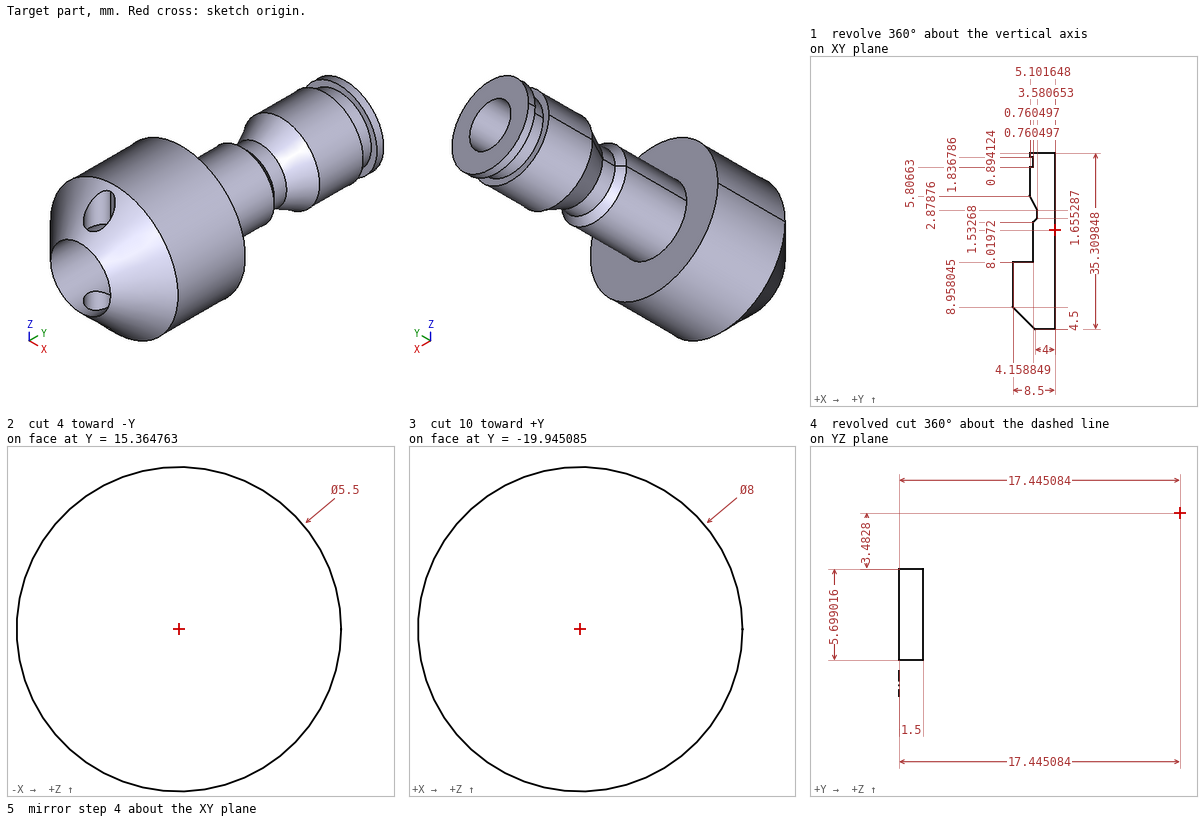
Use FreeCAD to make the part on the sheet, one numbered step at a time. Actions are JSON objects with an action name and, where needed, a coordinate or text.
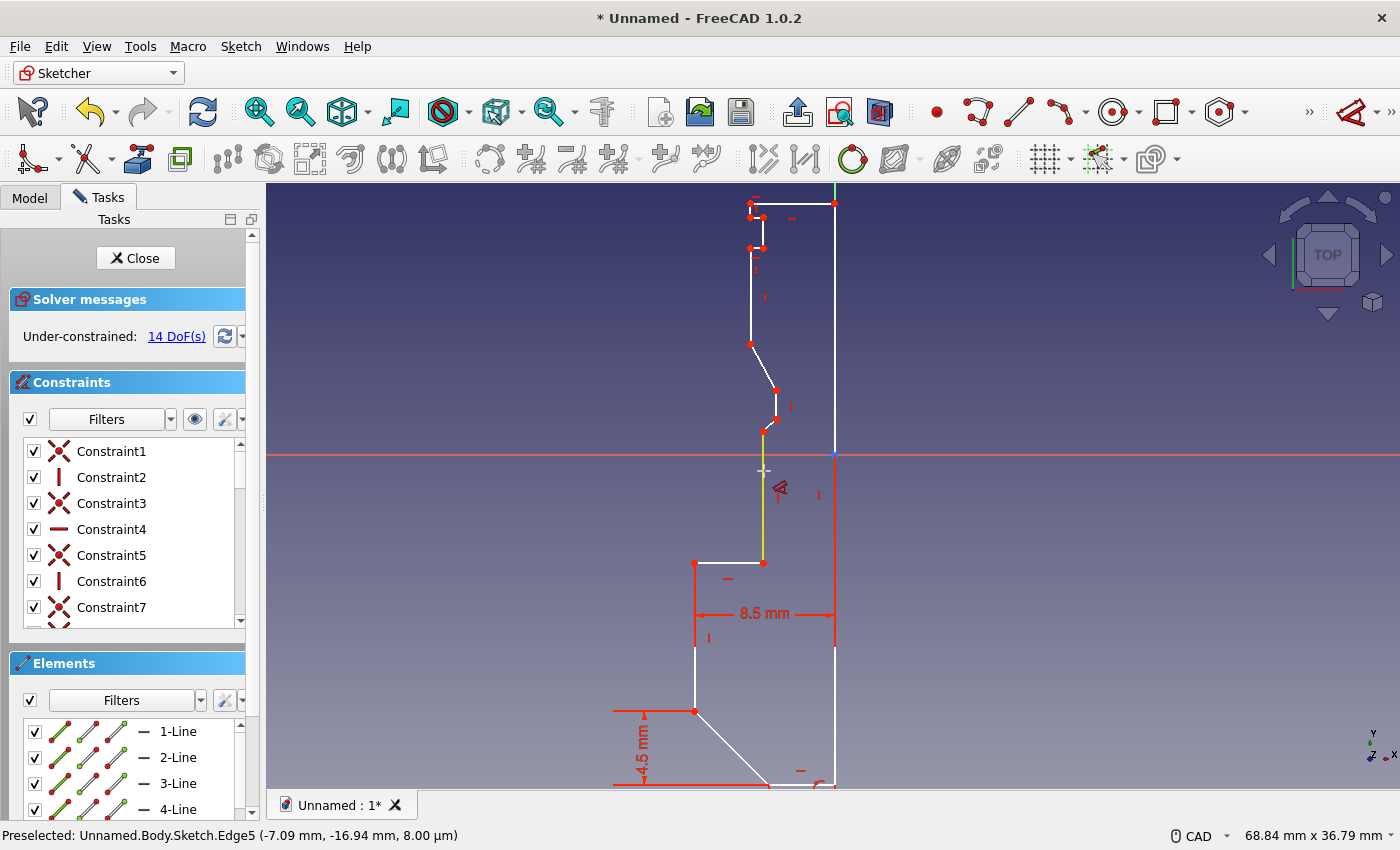
{"action": "left_click", "coordinate": [763, 471]}
{"action": "left_click", "coordinate": [729, 497]}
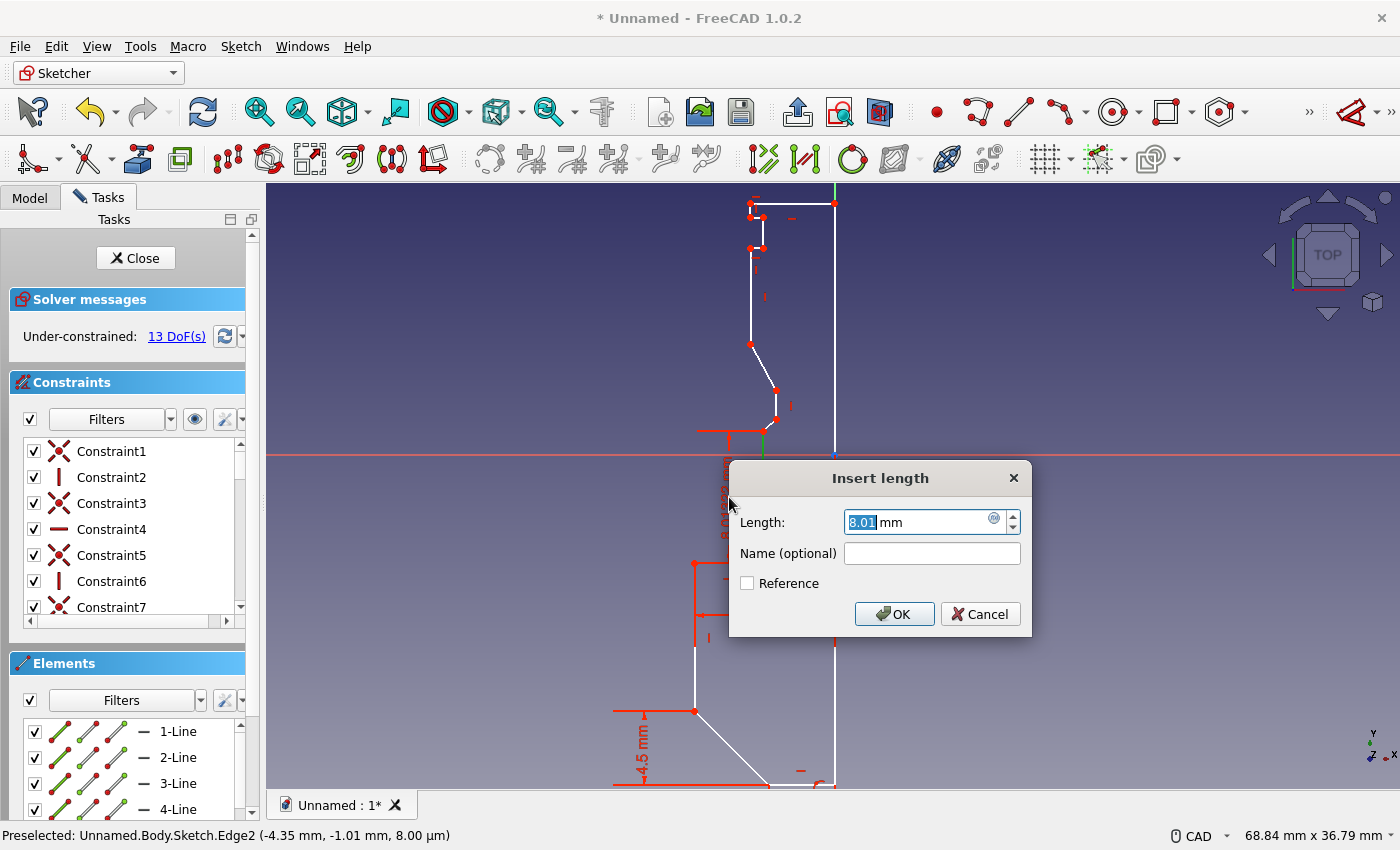
{"action": "type", "text": "8.01972"}
{"action": "key", "text": "Return"}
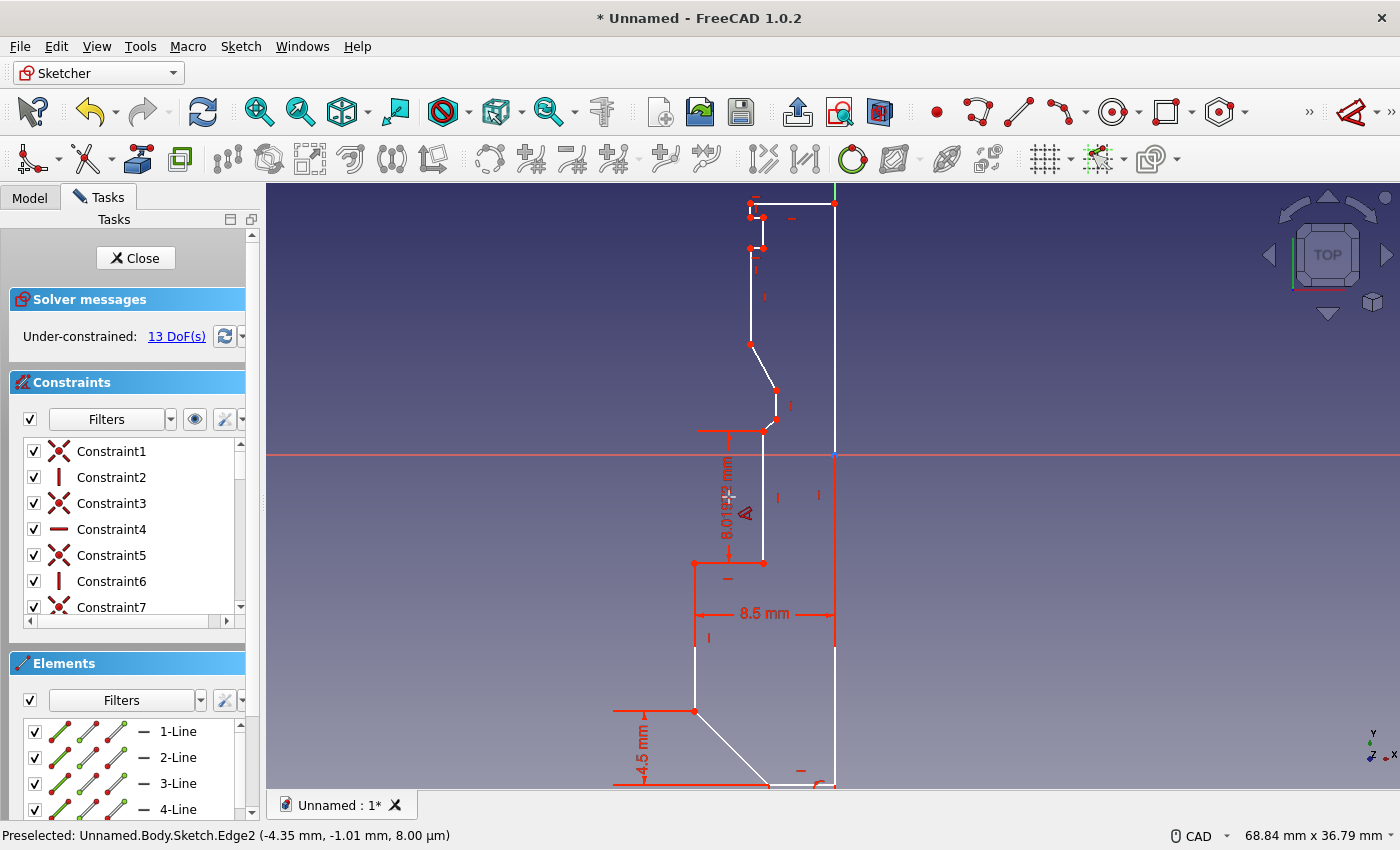
{"action": "left_click", "coordinate": [751, 277]}
{"action": "left_click", "coordinate": [717, 296]}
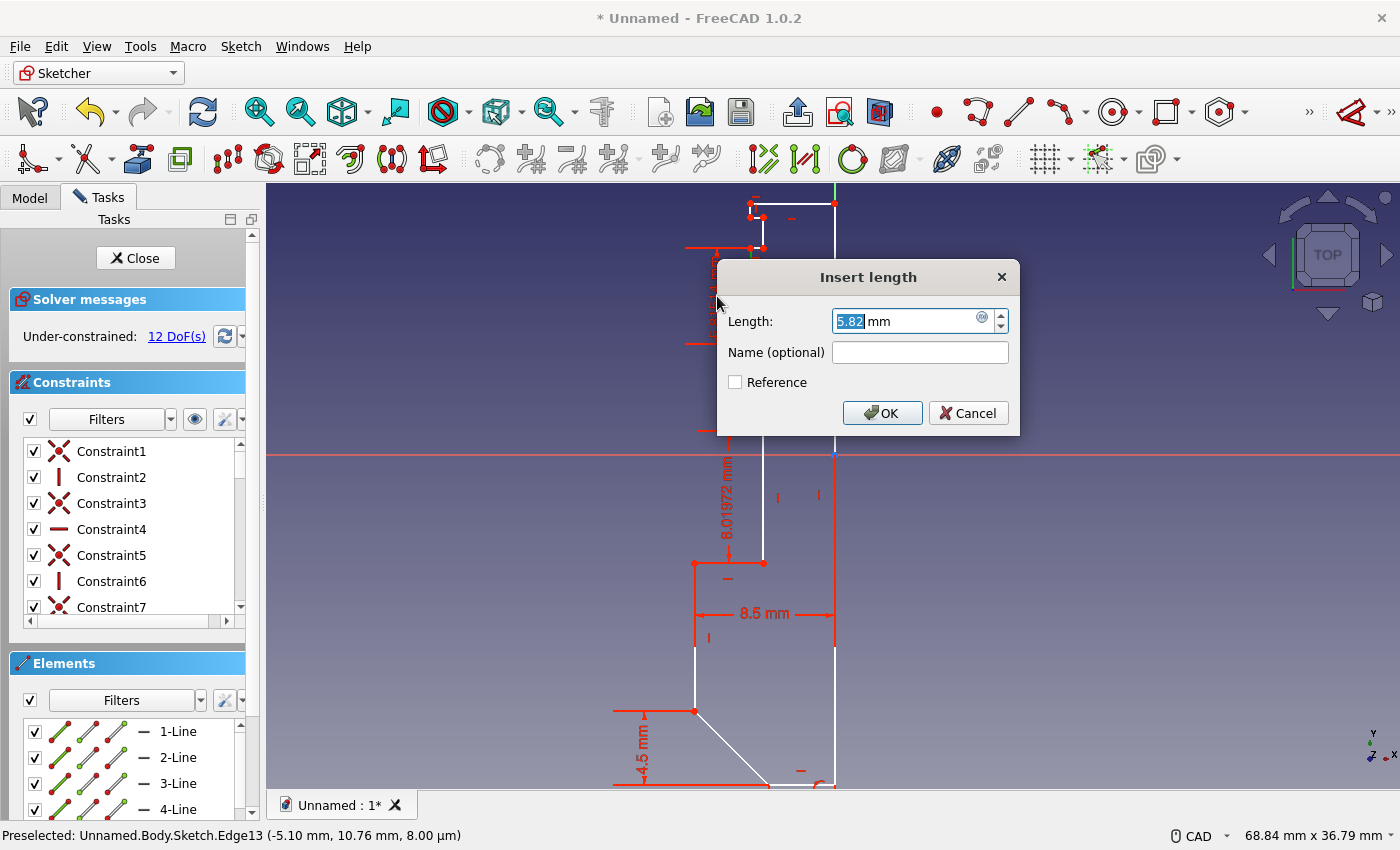
{"action": "type", "text": "5.80663"}
{"action": "key", "text": "Return"}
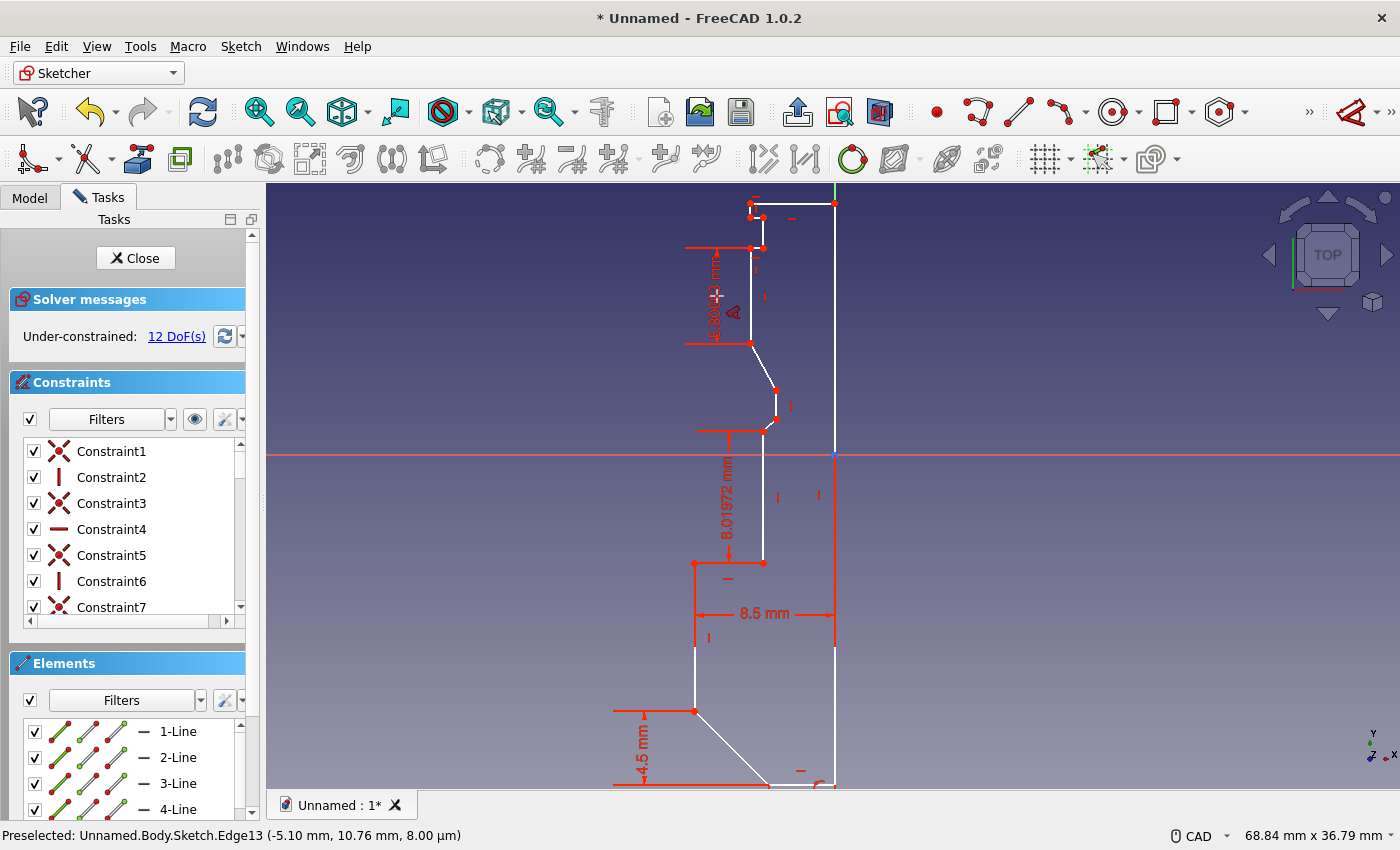
{"action": "left_click", "coordinate": [743, 563]}
{"action": "left_click", "coordinate": [729, 529]}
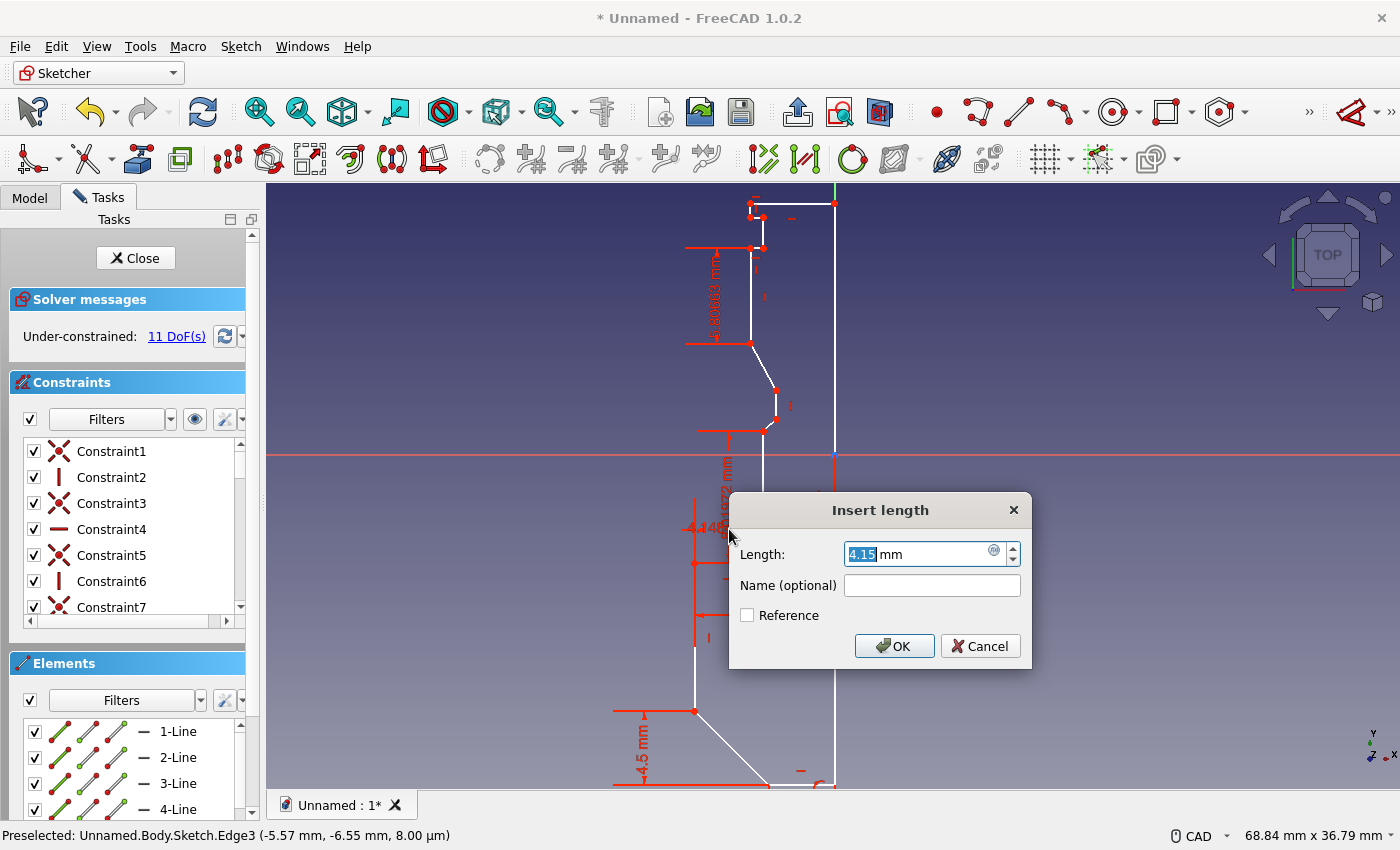
{"action": "type", "text": "4.158849"}
{"action": "key", "text": "Return"}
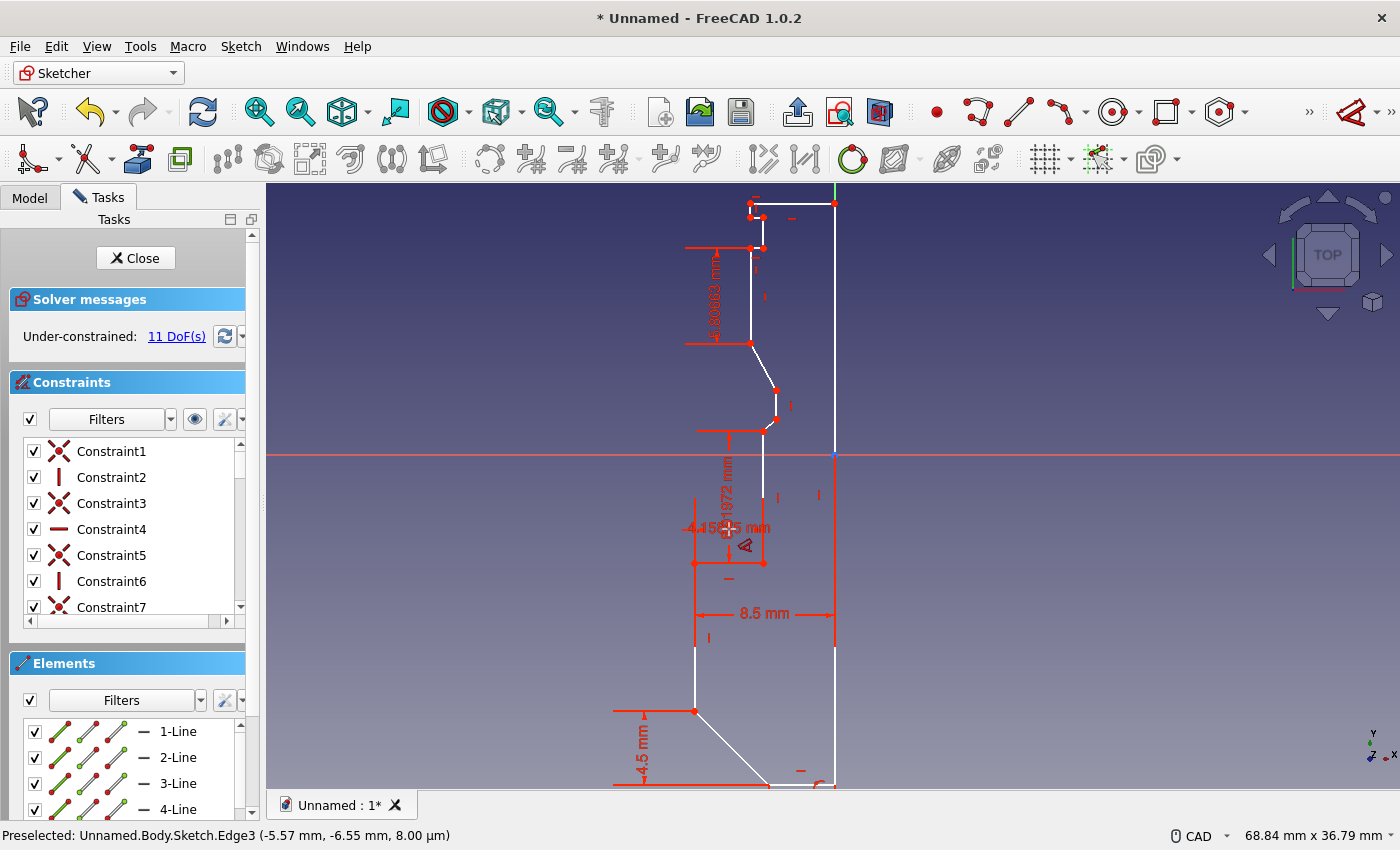
{"action": "left_click", "coordinate": [695, 608]}
{"action": "left_click", "coordinate": [661, 637]}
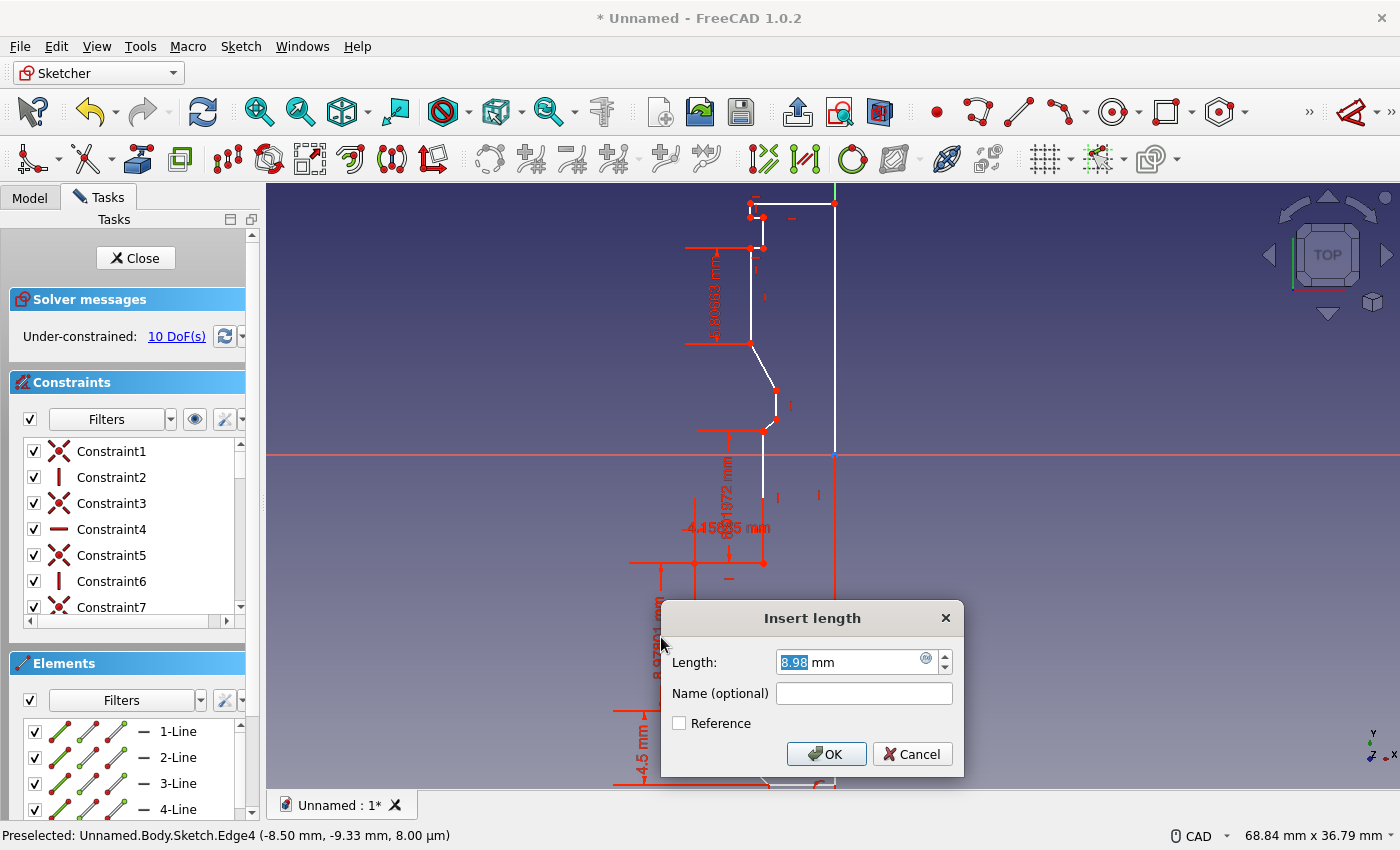
{"action": "type", "text": "8.958045"}
{"action": "key", "text": "Return"}